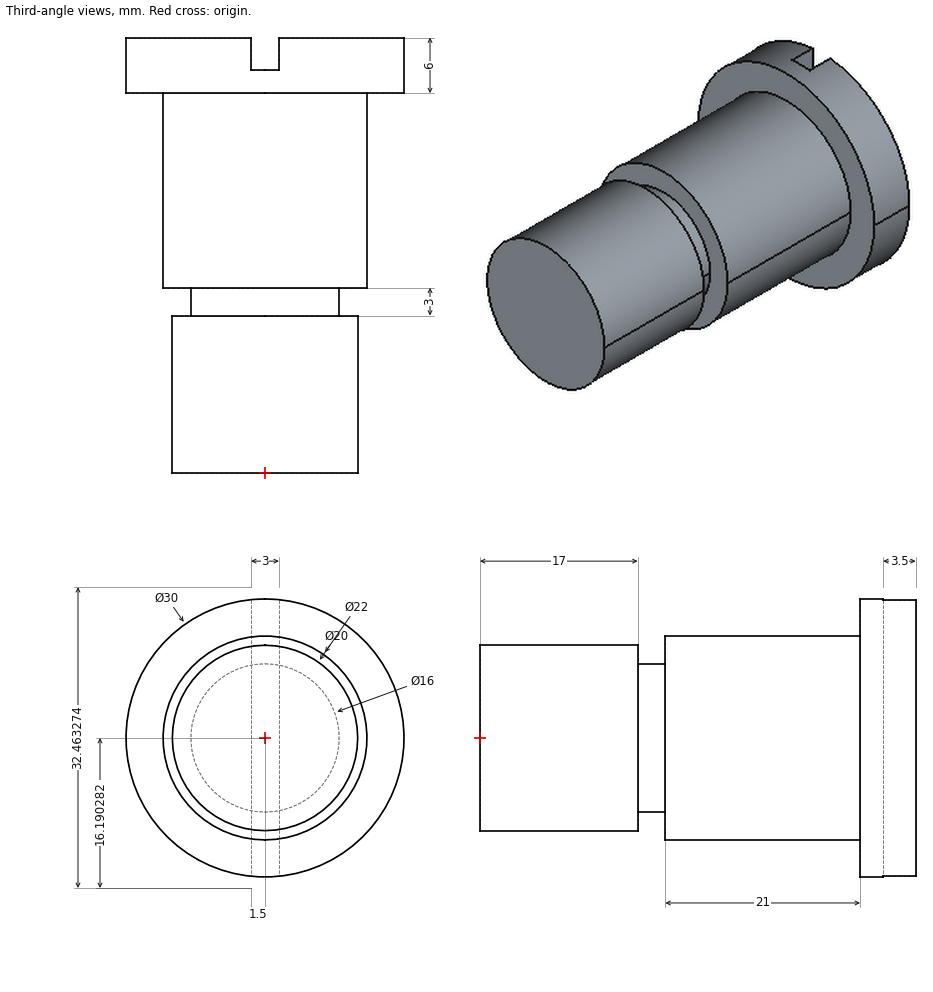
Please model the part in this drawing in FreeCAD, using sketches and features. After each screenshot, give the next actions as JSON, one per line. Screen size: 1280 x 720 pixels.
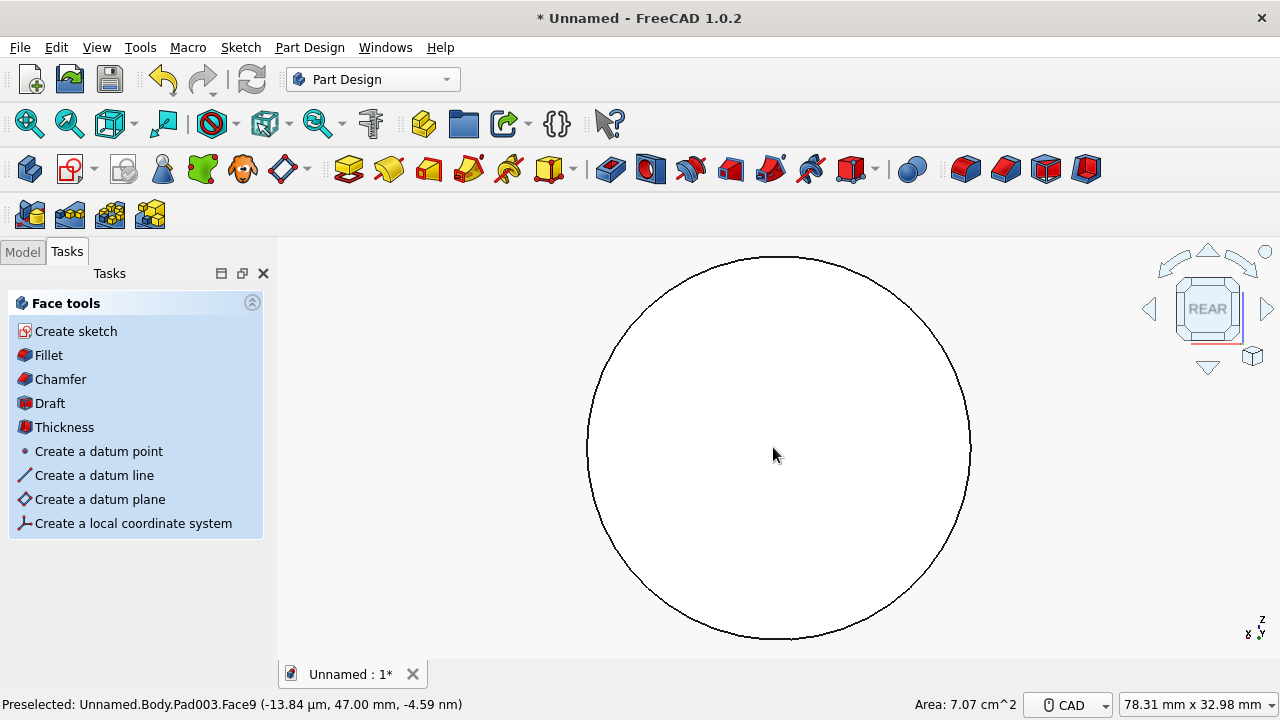
{"action": "left_click", "coordinate": [70, 170]}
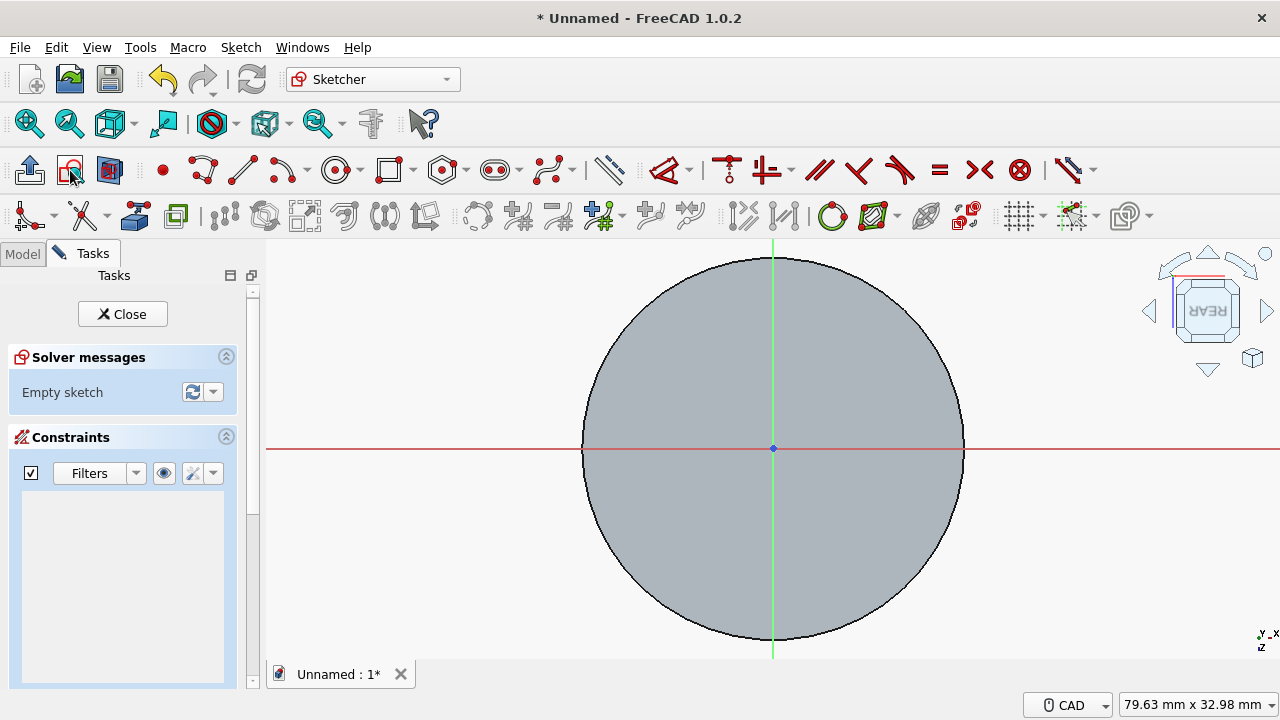
{"action": "scroll", "coordinate": [565, 448], "scroll_direction": "down", "scroll_amount": 2}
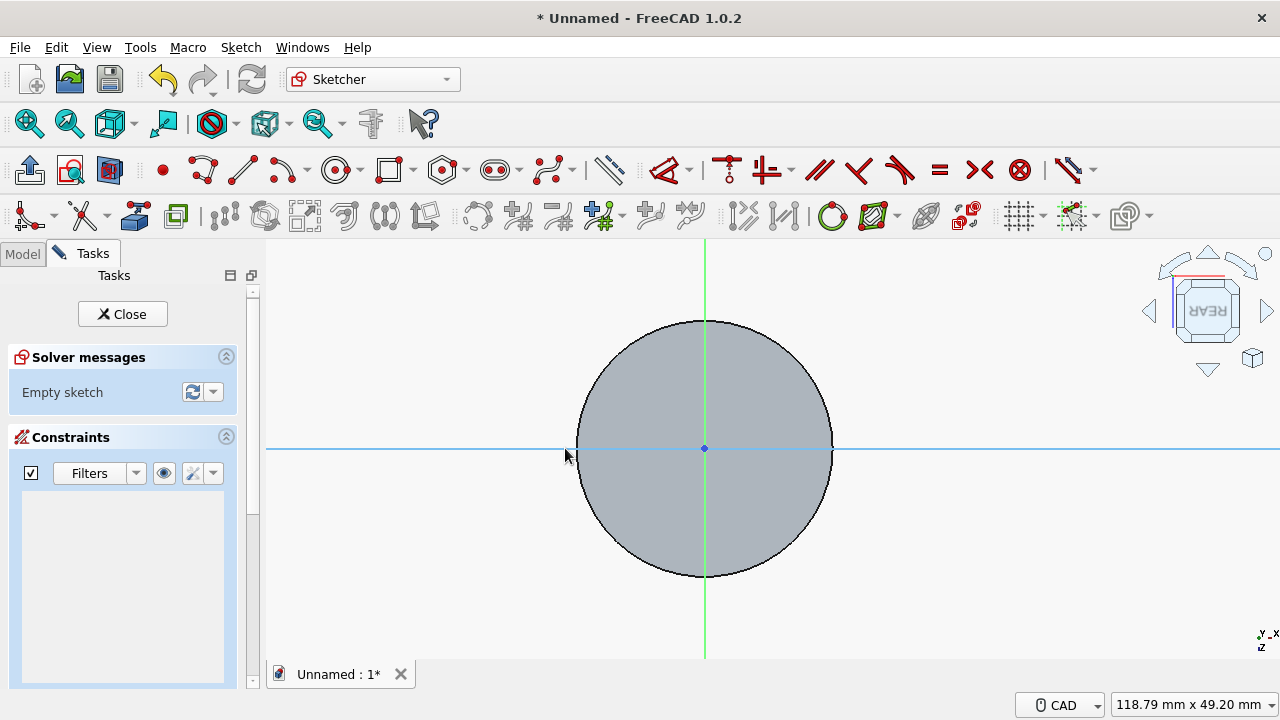
{"action": "key", "text": "g r"}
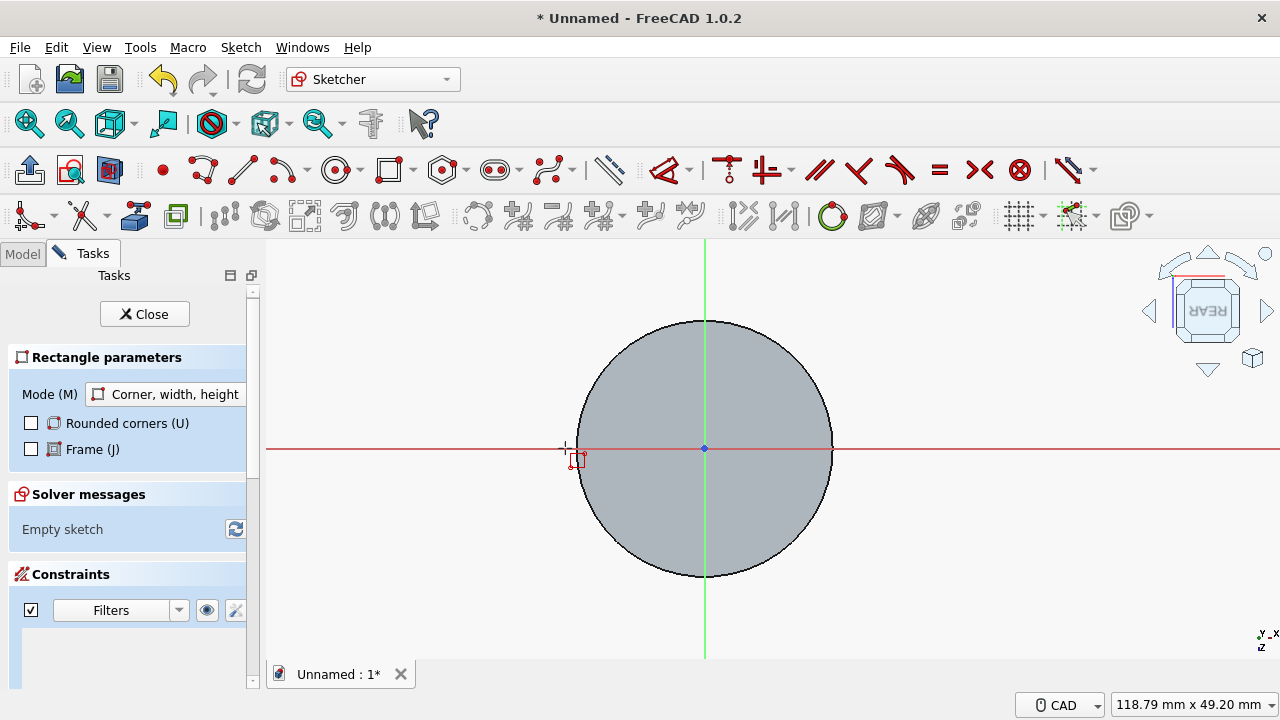
{"action": "scroll", "coordinate": [692, 311], "scroll_direction": "up", "scroll_amount": 2}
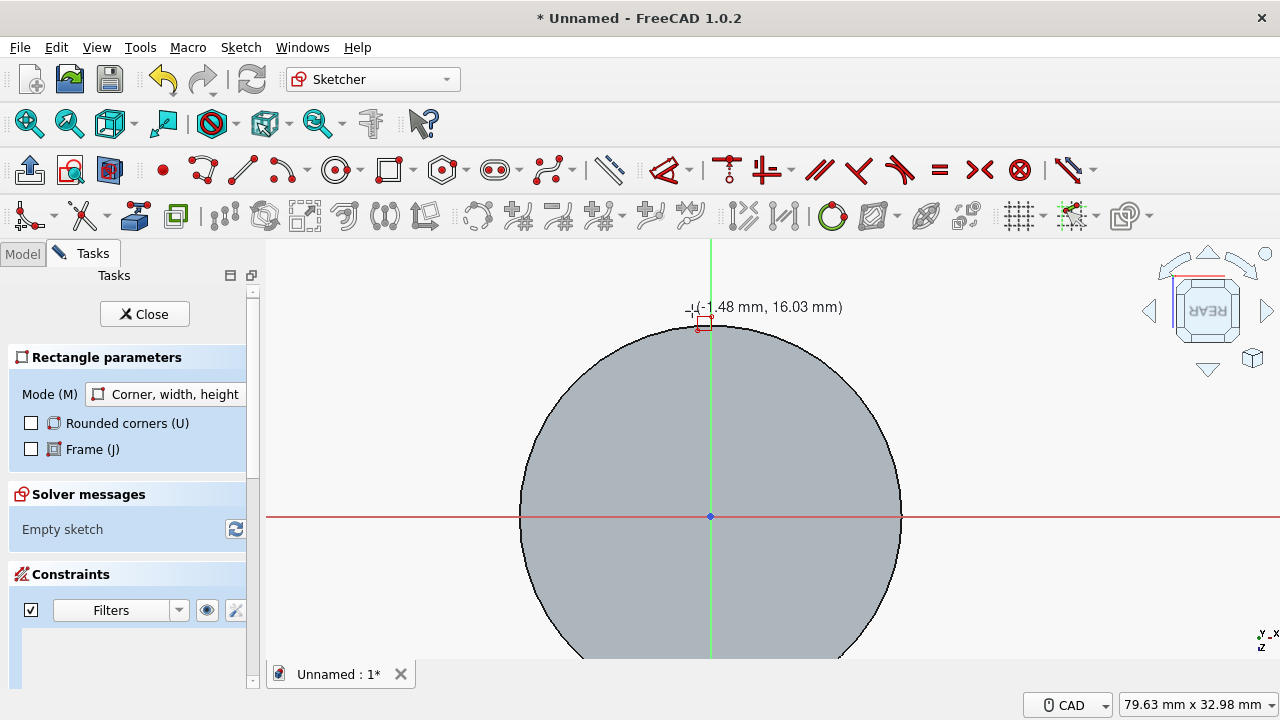
{"action": "left_click", "coordinate": [692, 310]}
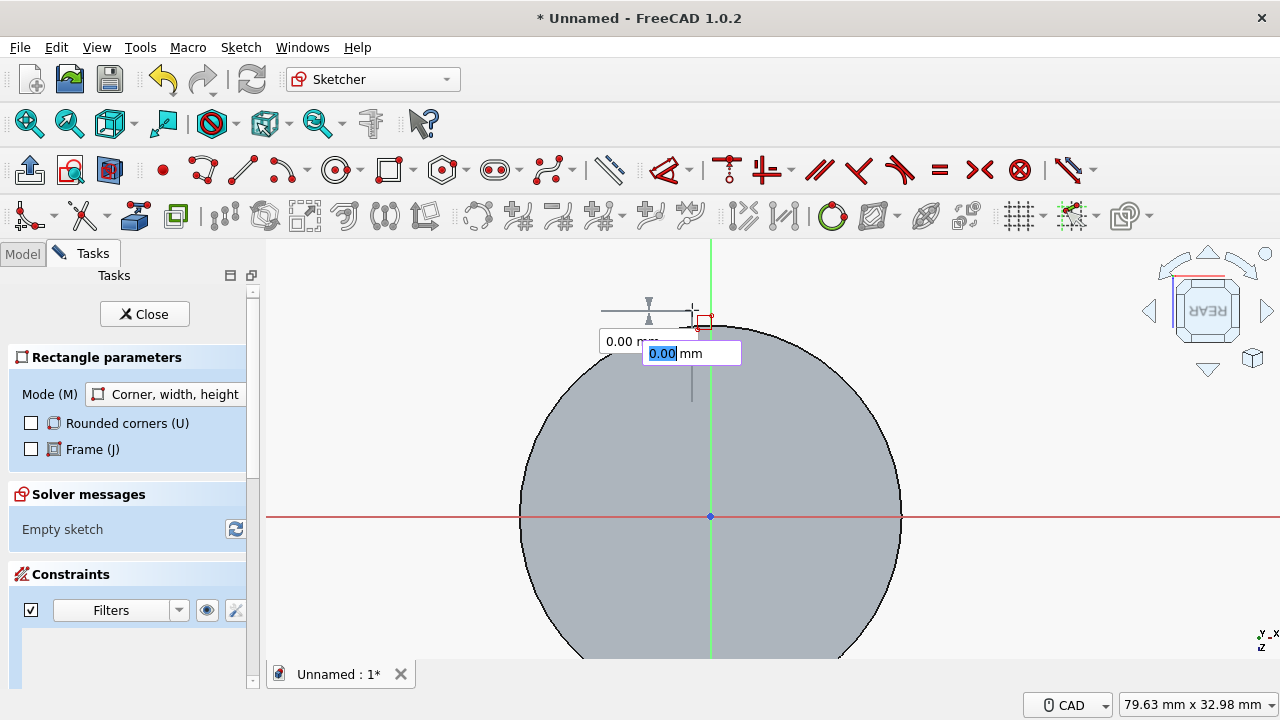
{"action": "scroll", "coordinate": [692, 311], "scroll_direction": "down", "scroll_amount": 2}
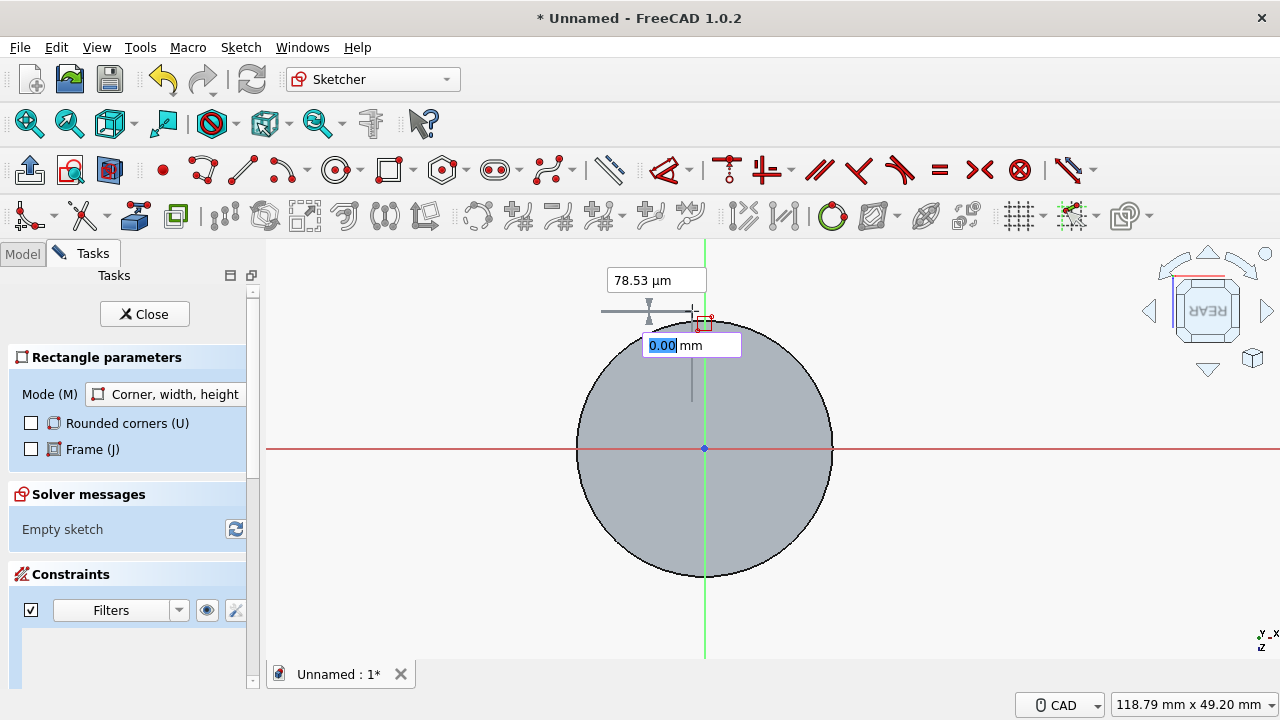
{"action": "scroll", "coordinate": [717, 588], "scroll_direction": "up", "scroll_amount": 2}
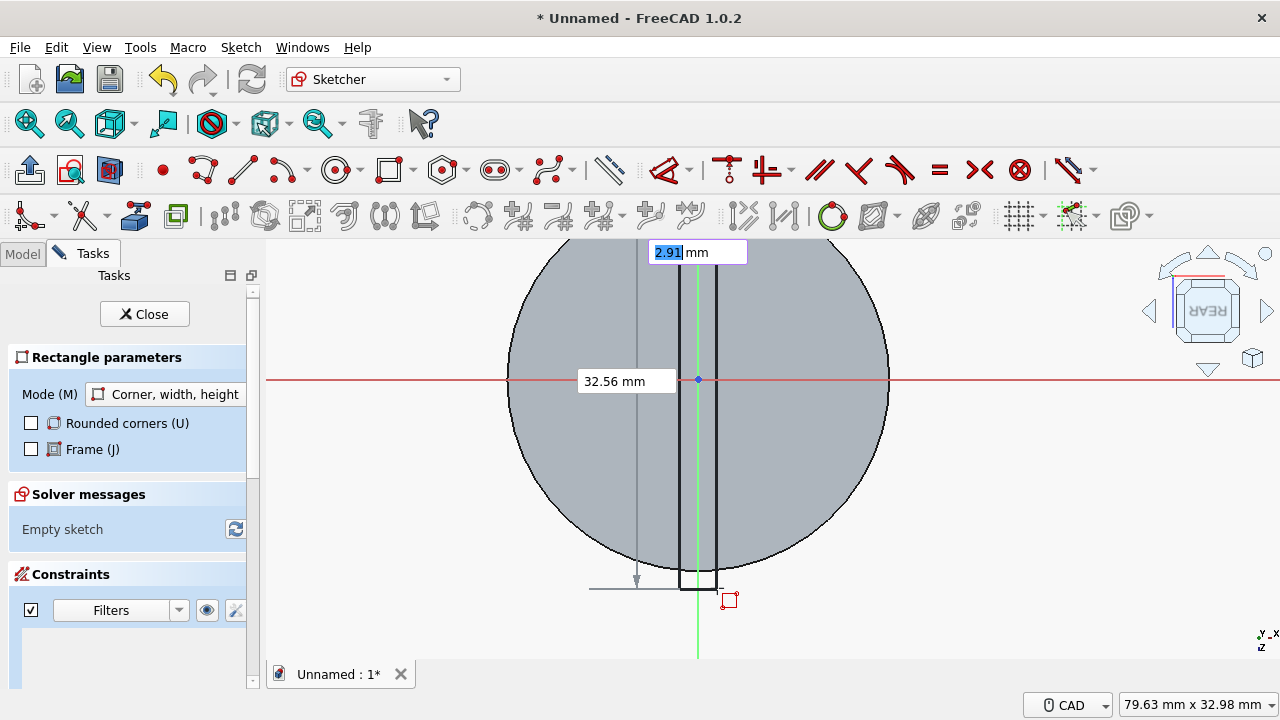
{"action": "left_click", "coordinate": [717, 587]}
{"action": "key", "text": "Escape"}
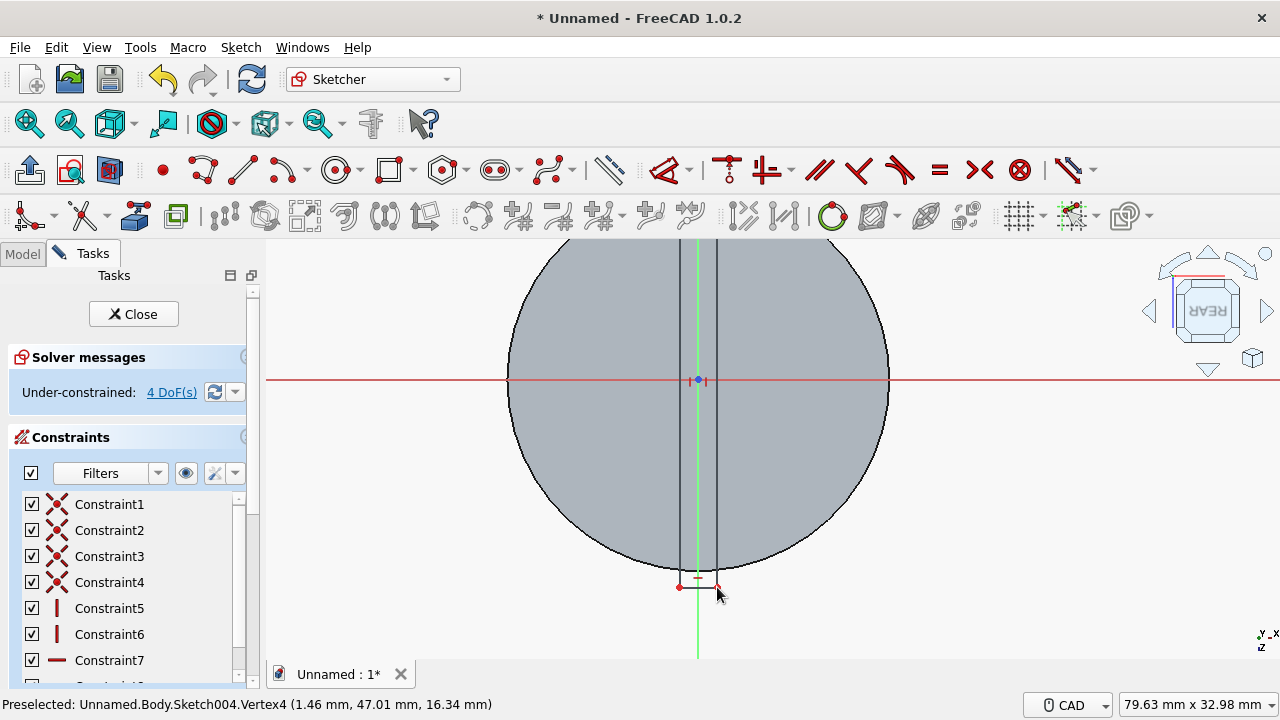
{"action": "left_click", "coordinate": [664, 170]}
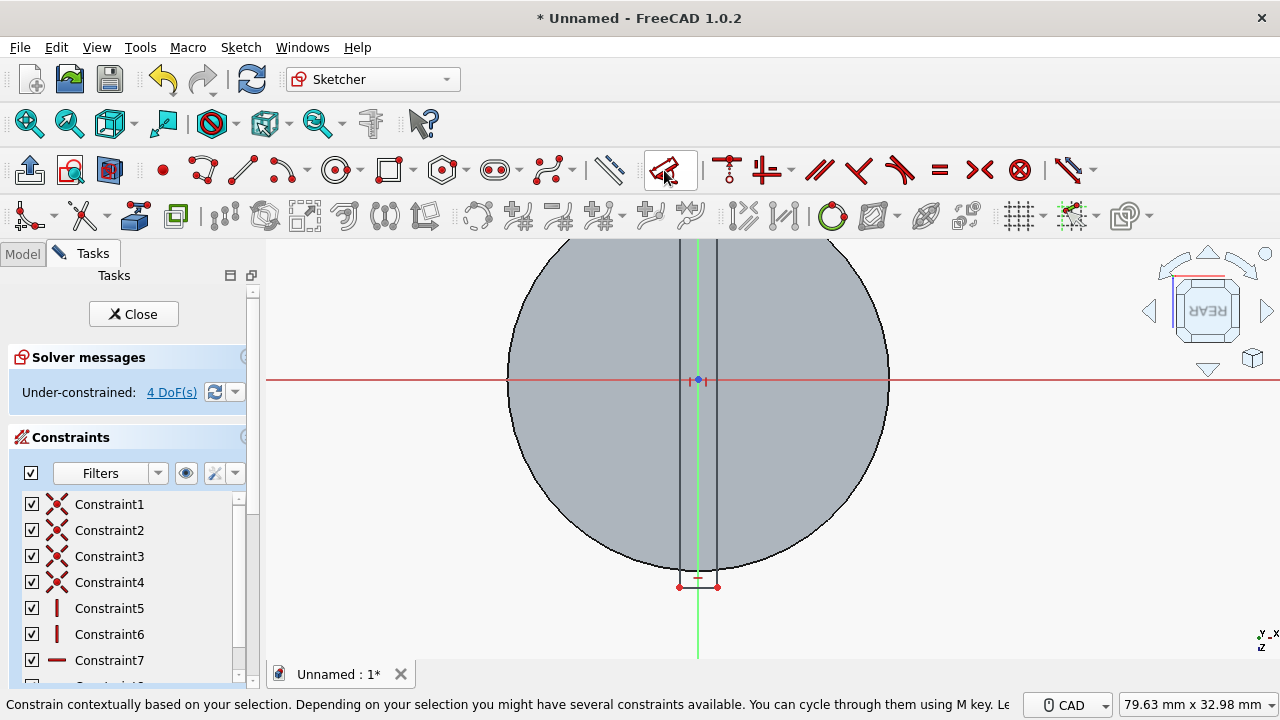
{"action": "left_click", "coordinate": [695, 588]}
{"action": "left_click", "coordinate": [685, 622]}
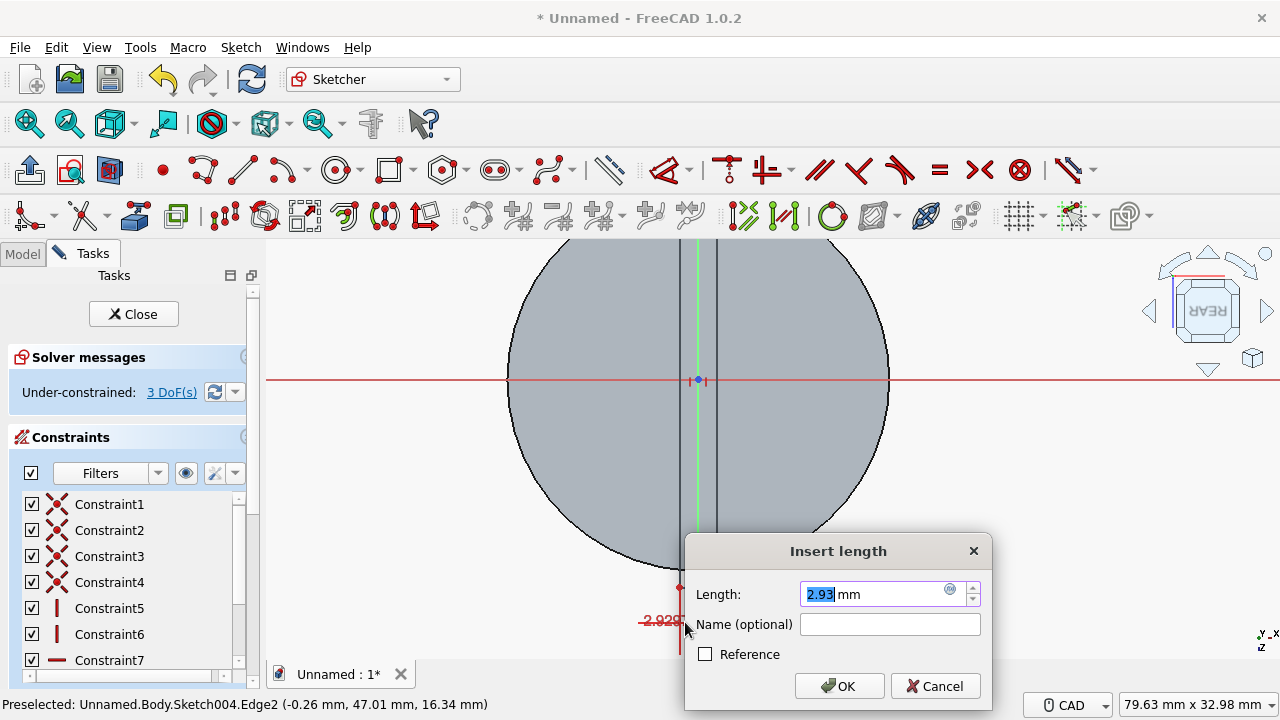
{"action": "type", "text": "3"}
{"action": "key", "text": "Return"}